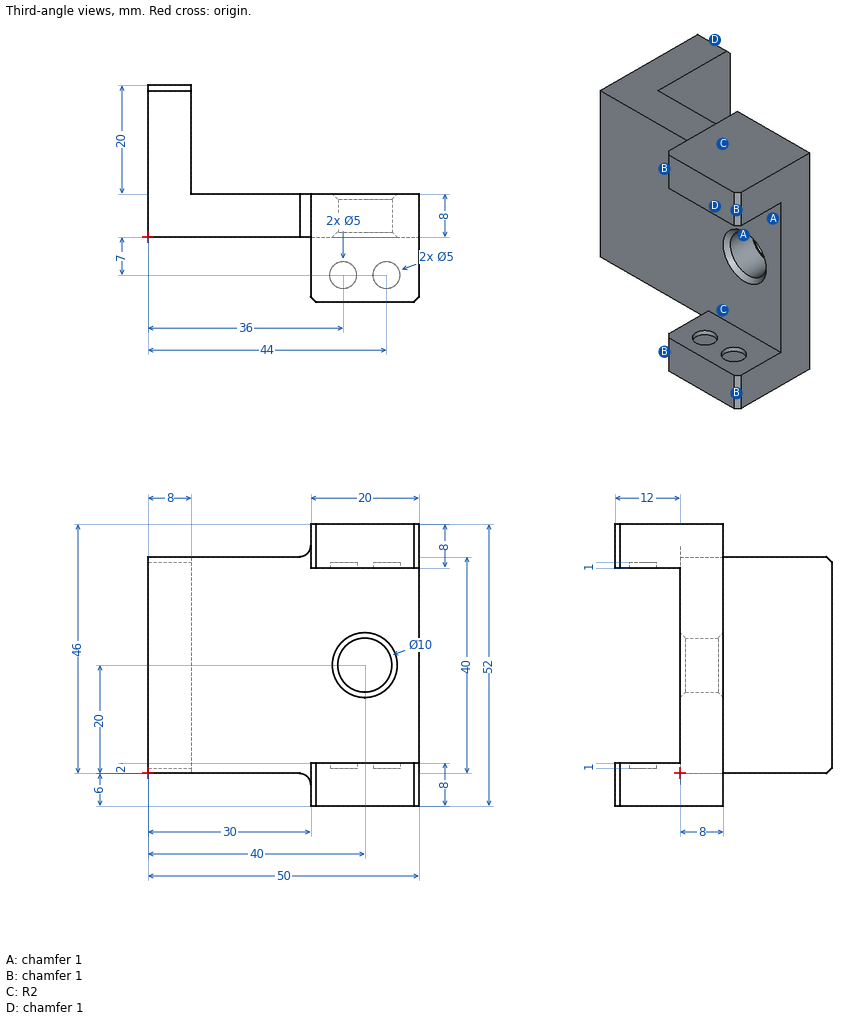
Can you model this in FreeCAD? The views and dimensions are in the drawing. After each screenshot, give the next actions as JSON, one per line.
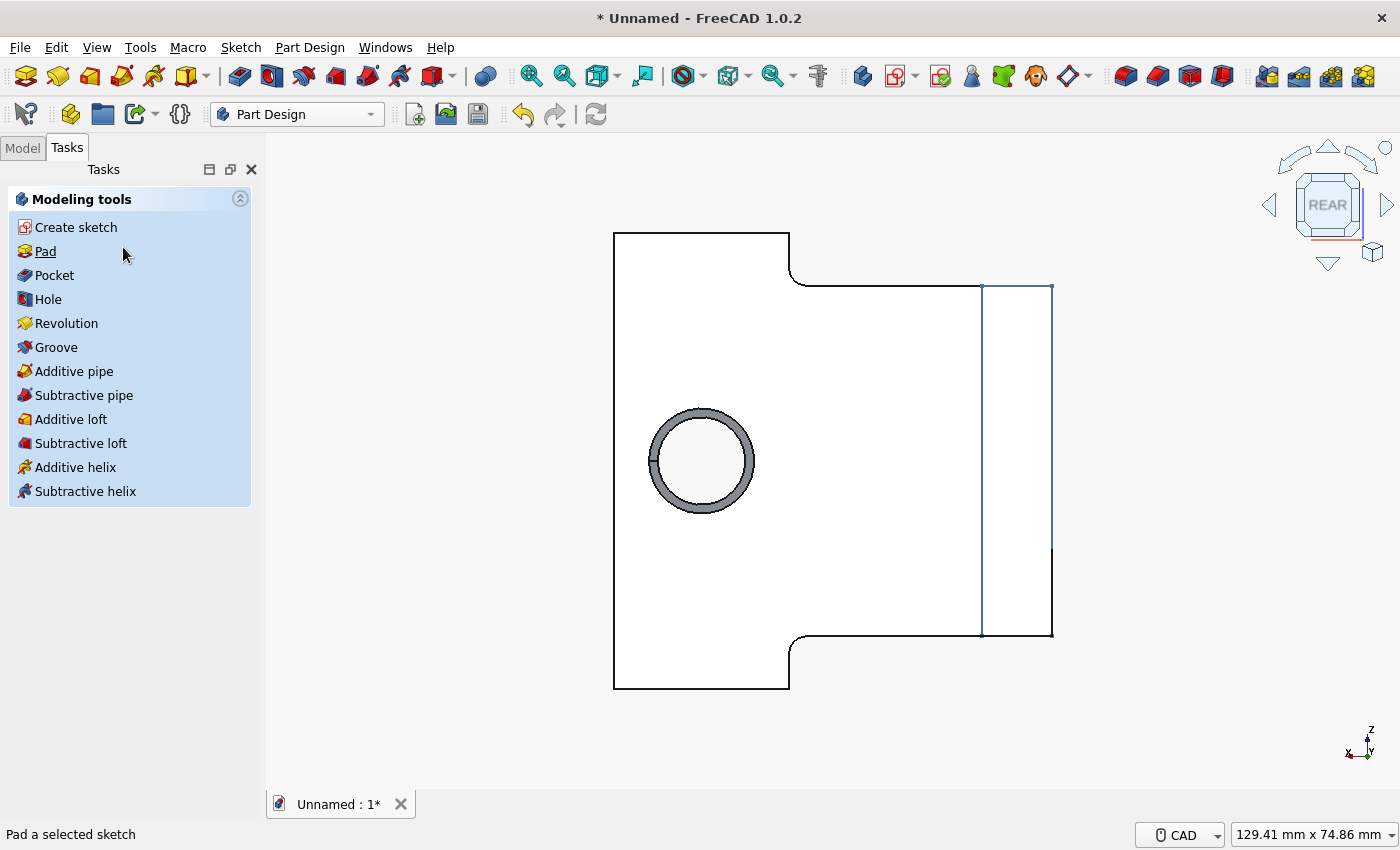
{"action": "left_click", "coordinate": [26, 76]}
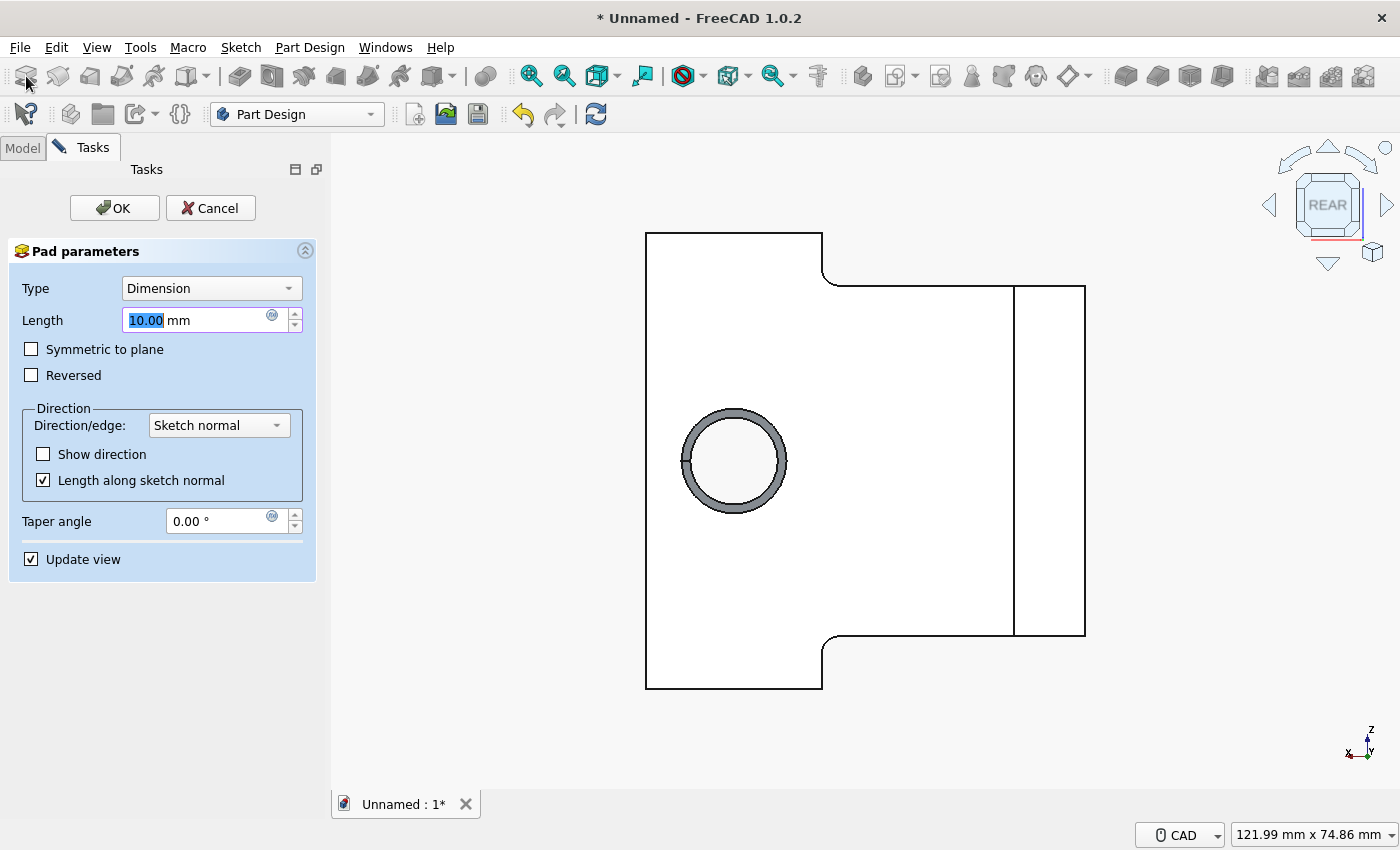
{"action": "type", "text": "20"}
{"action": "key", "text": "Tab"}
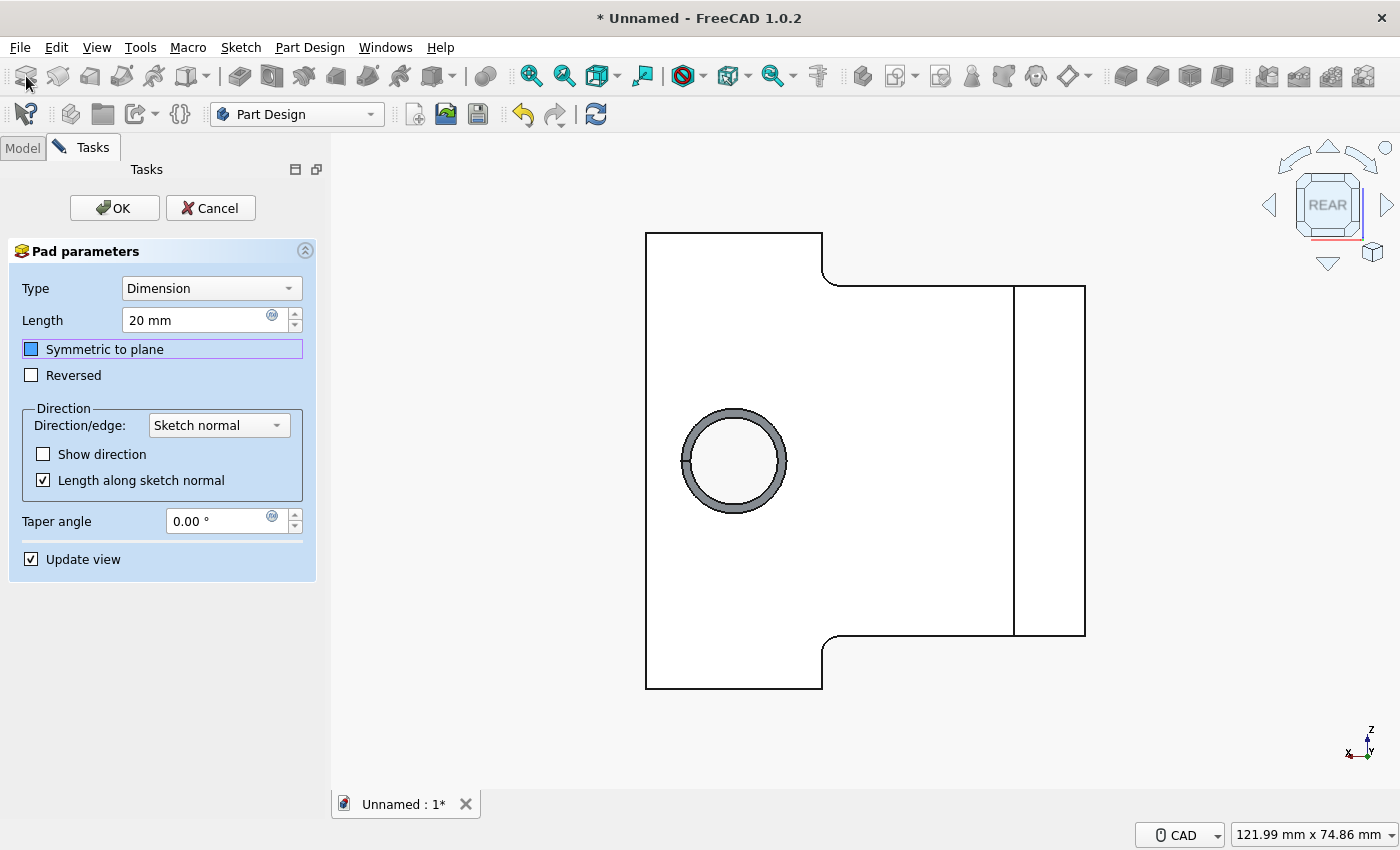
{"action": "left_click", "coordinate": [115, 208]}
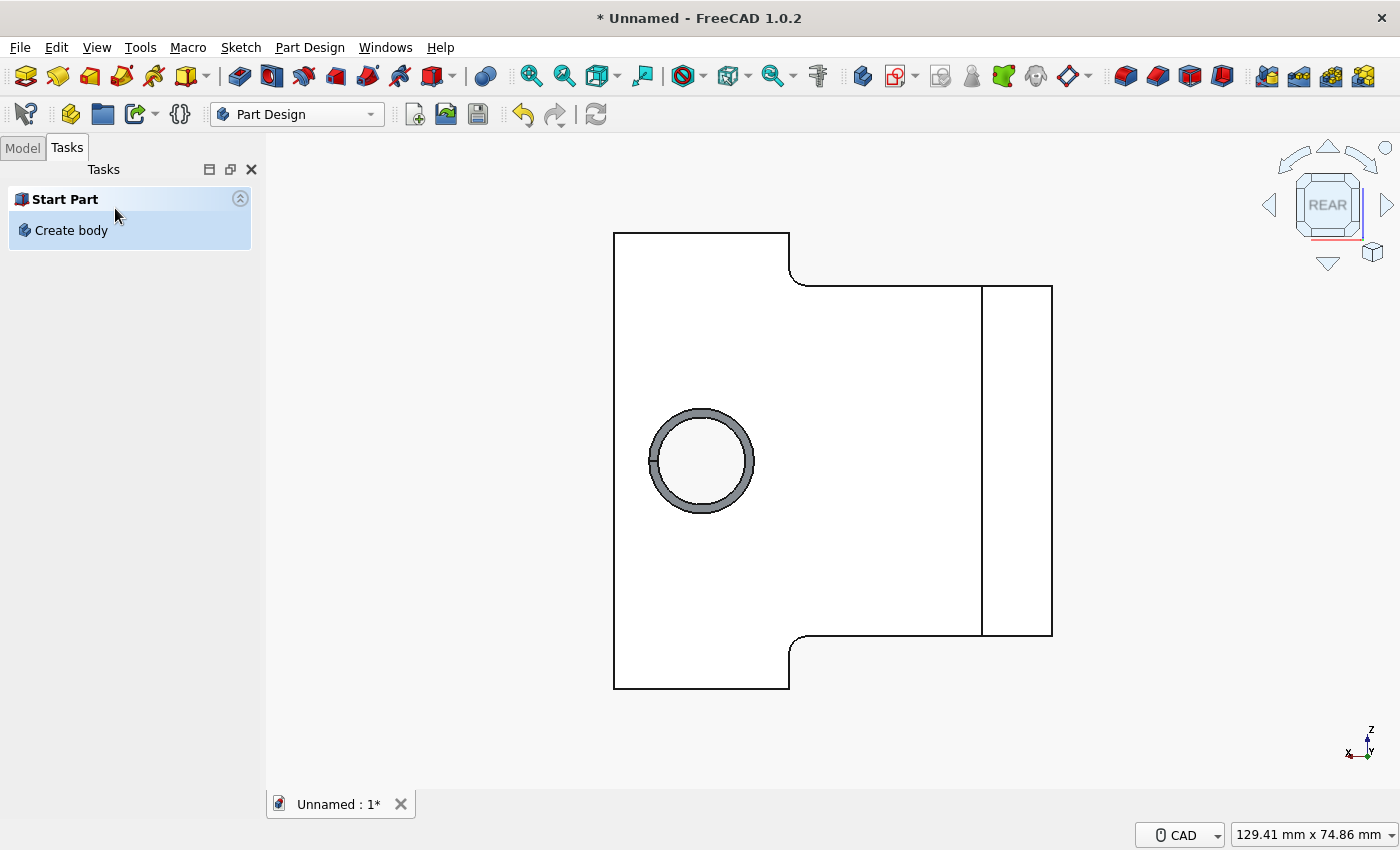
{"action": "left_click", "coordinate": [1017, 635]}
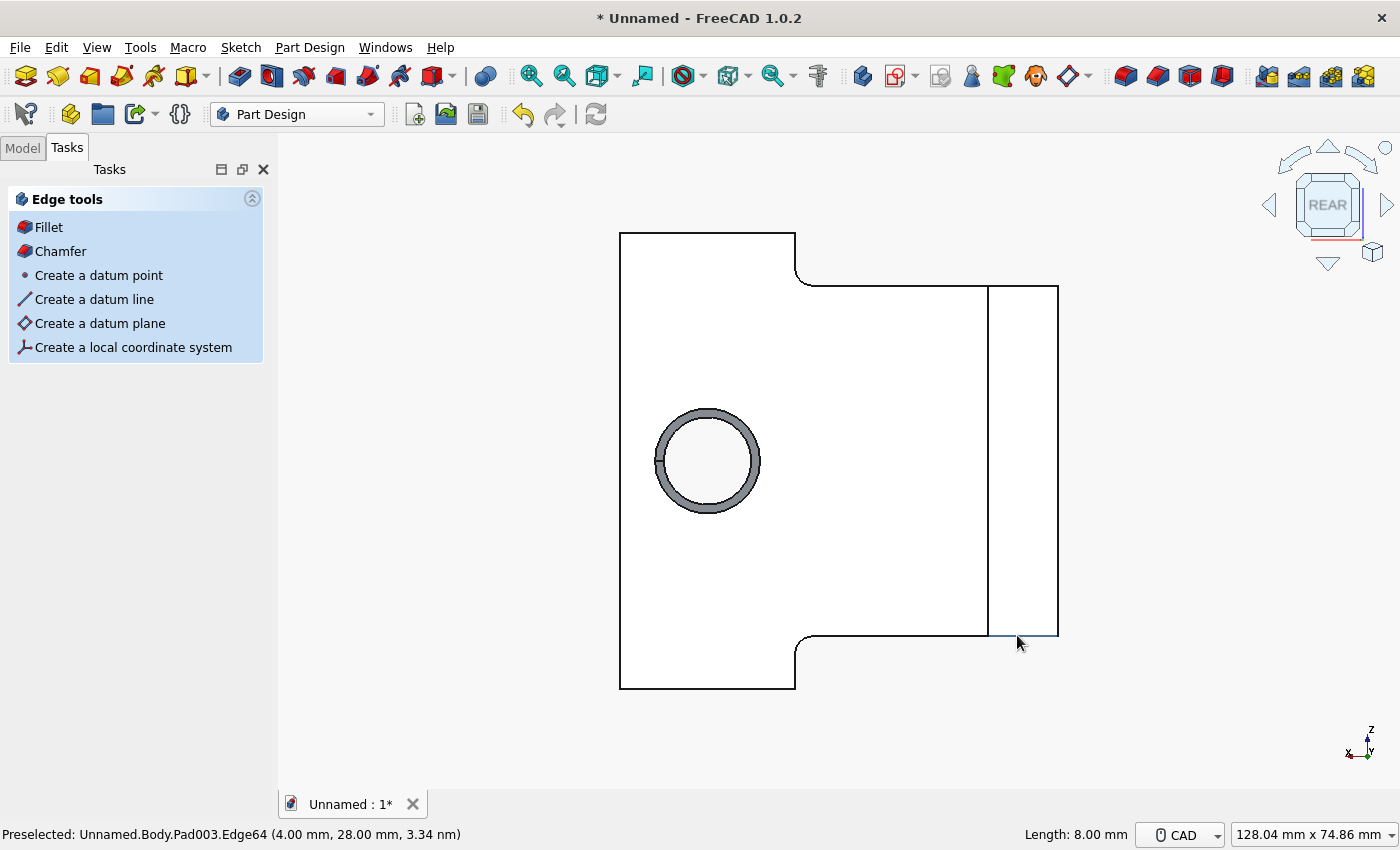
{"action": "key", "text": "0"}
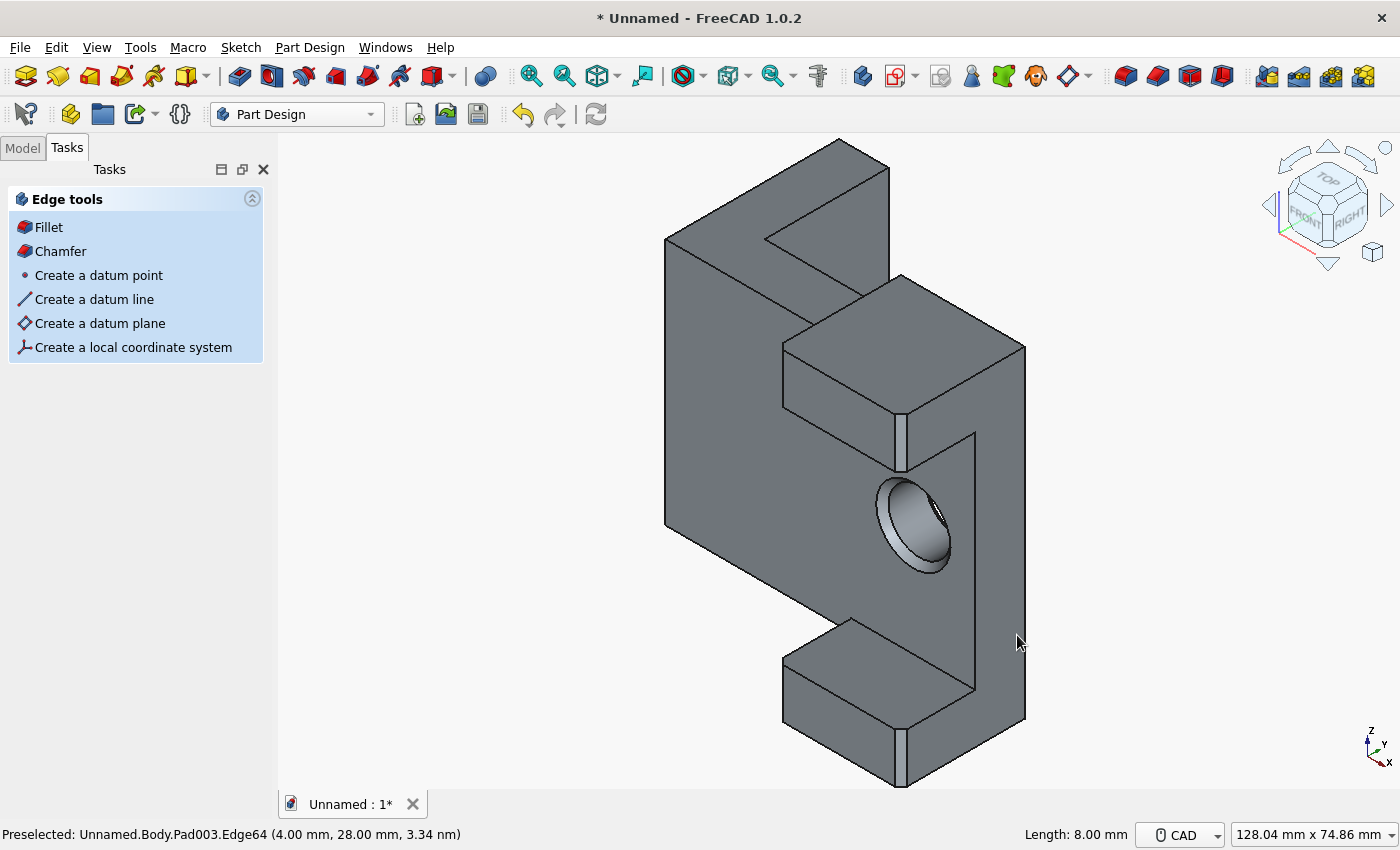
{"action": "left_click", "coordinate": [532, 76]}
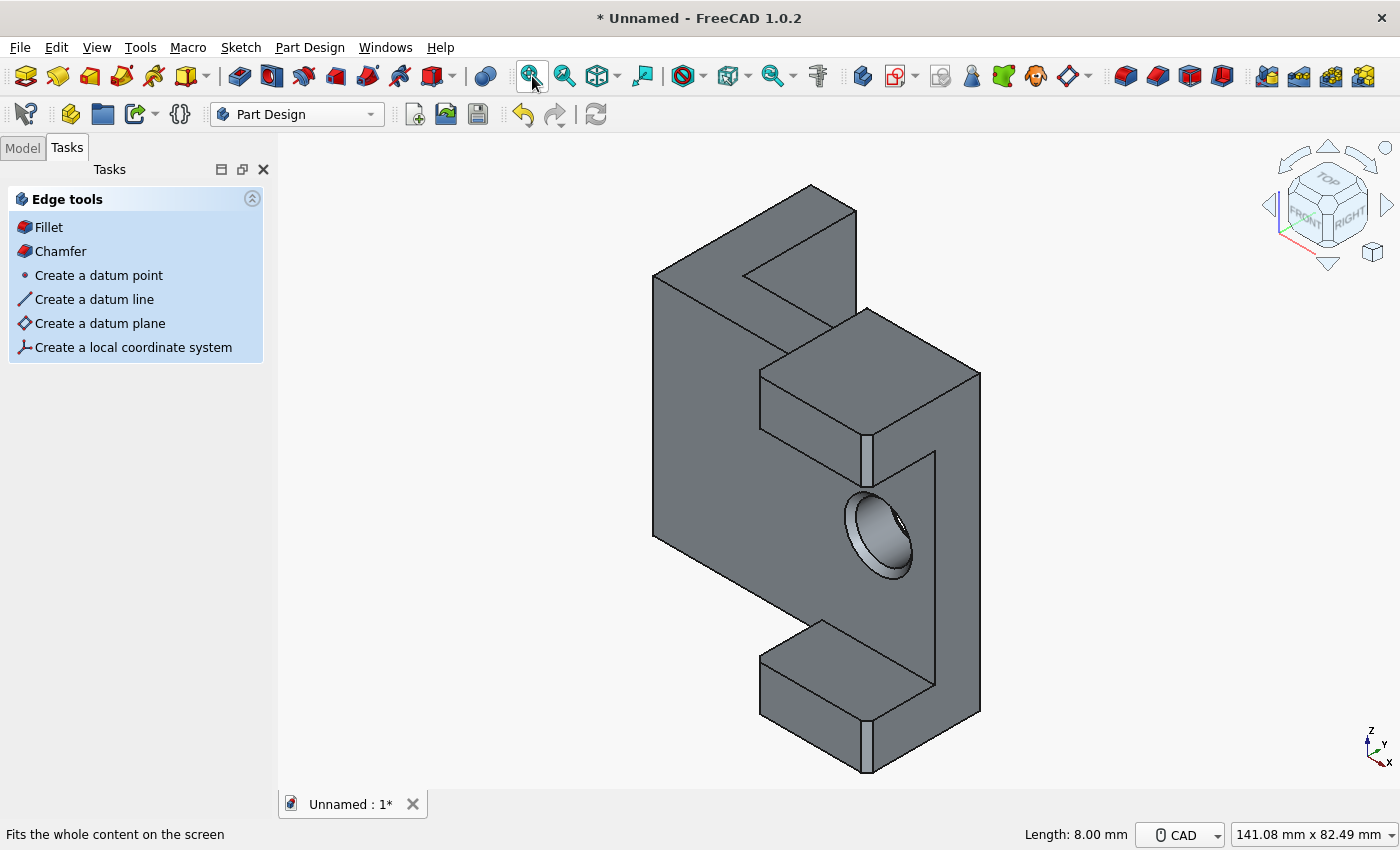
{"action": "key", "text": "2"}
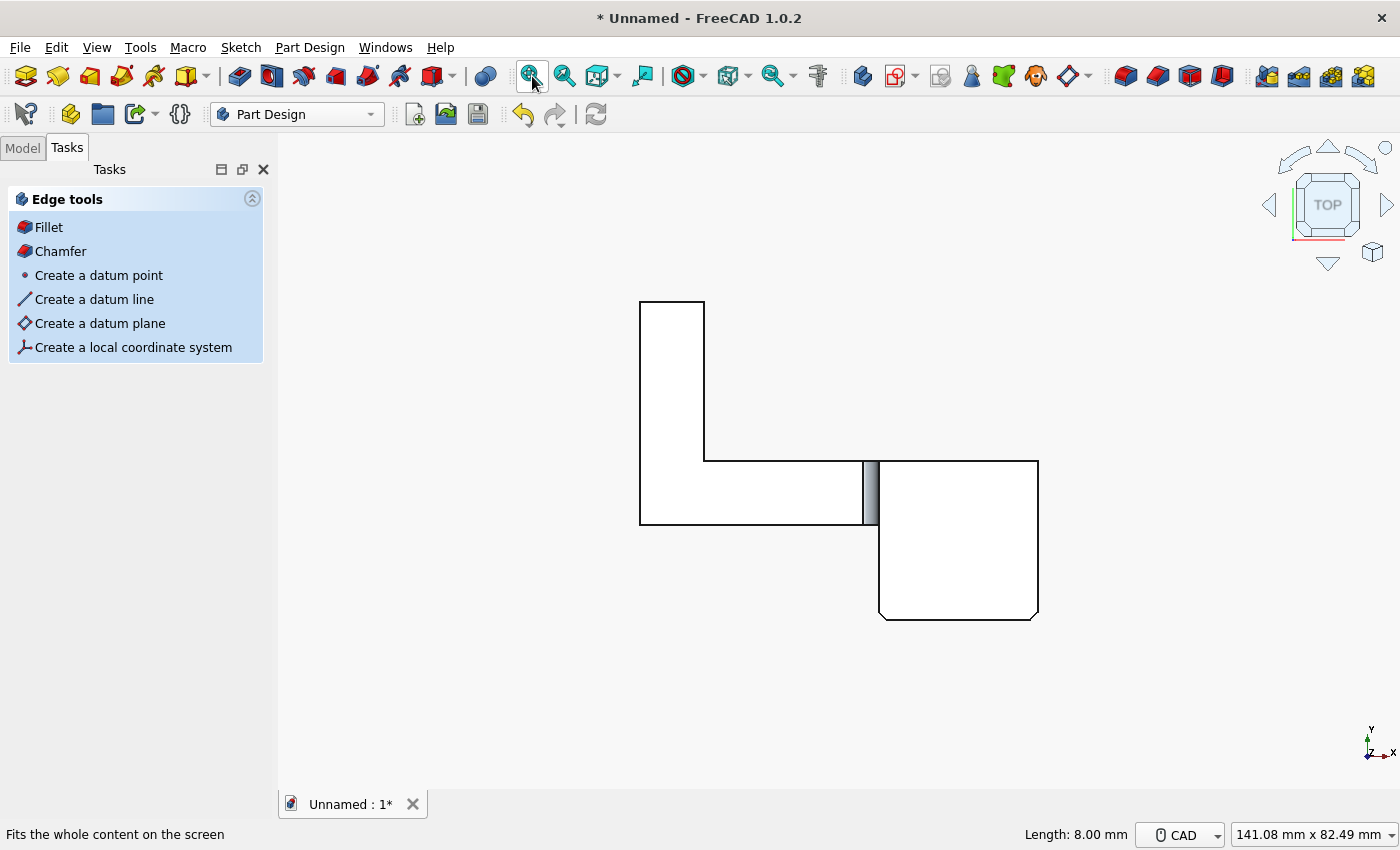
{"action": "left_click", "coordinate": [672, 301], "text": "ctrl"}